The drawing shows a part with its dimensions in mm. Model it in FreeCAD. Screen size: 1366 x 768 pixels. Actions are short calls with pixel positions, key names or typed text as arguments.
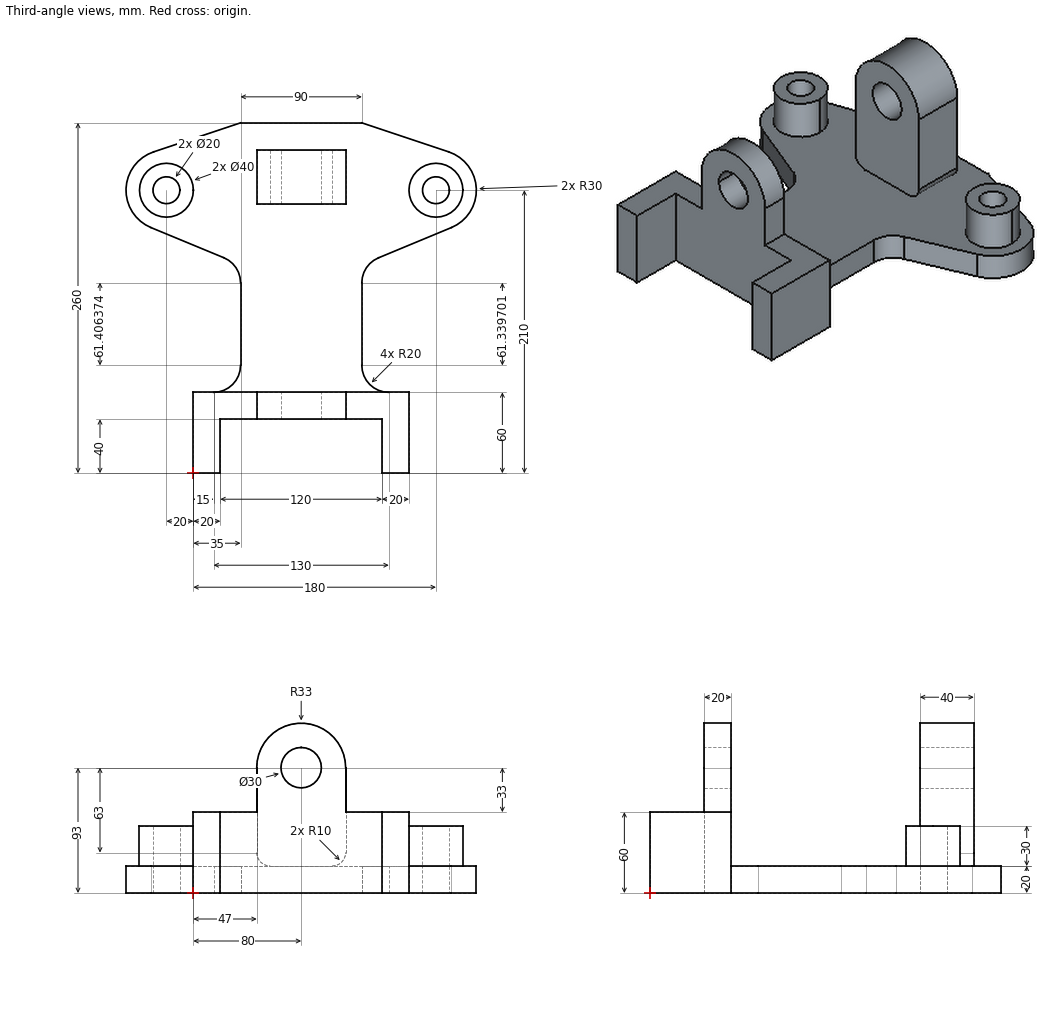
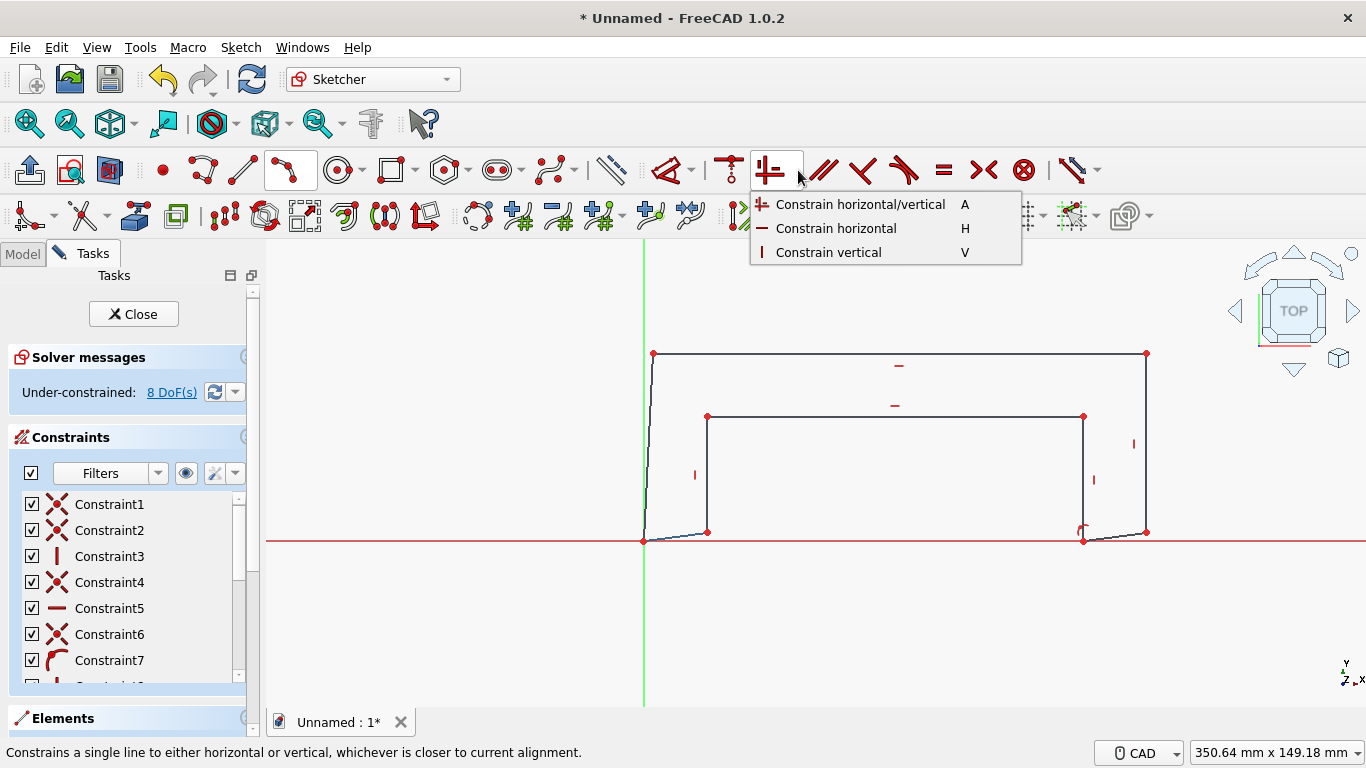
click(886, 228)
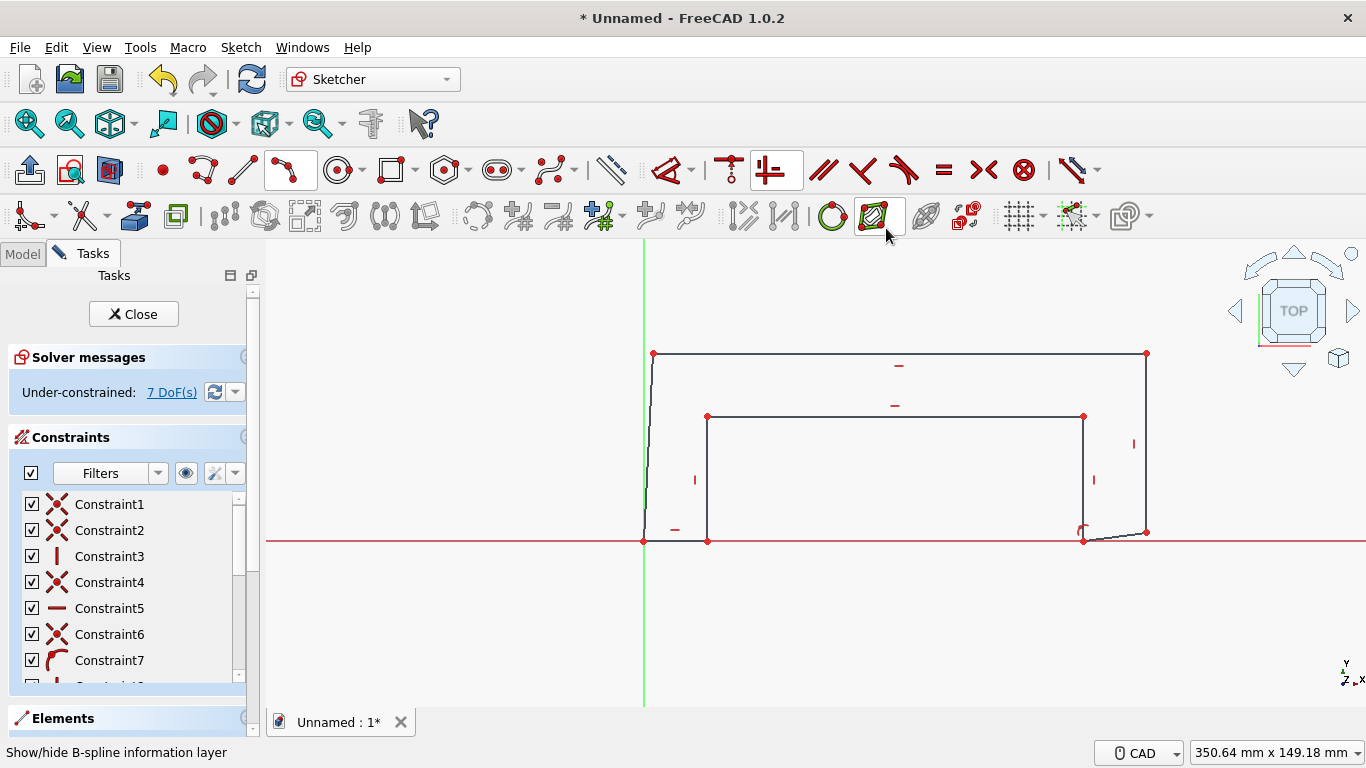
click(1102, 539)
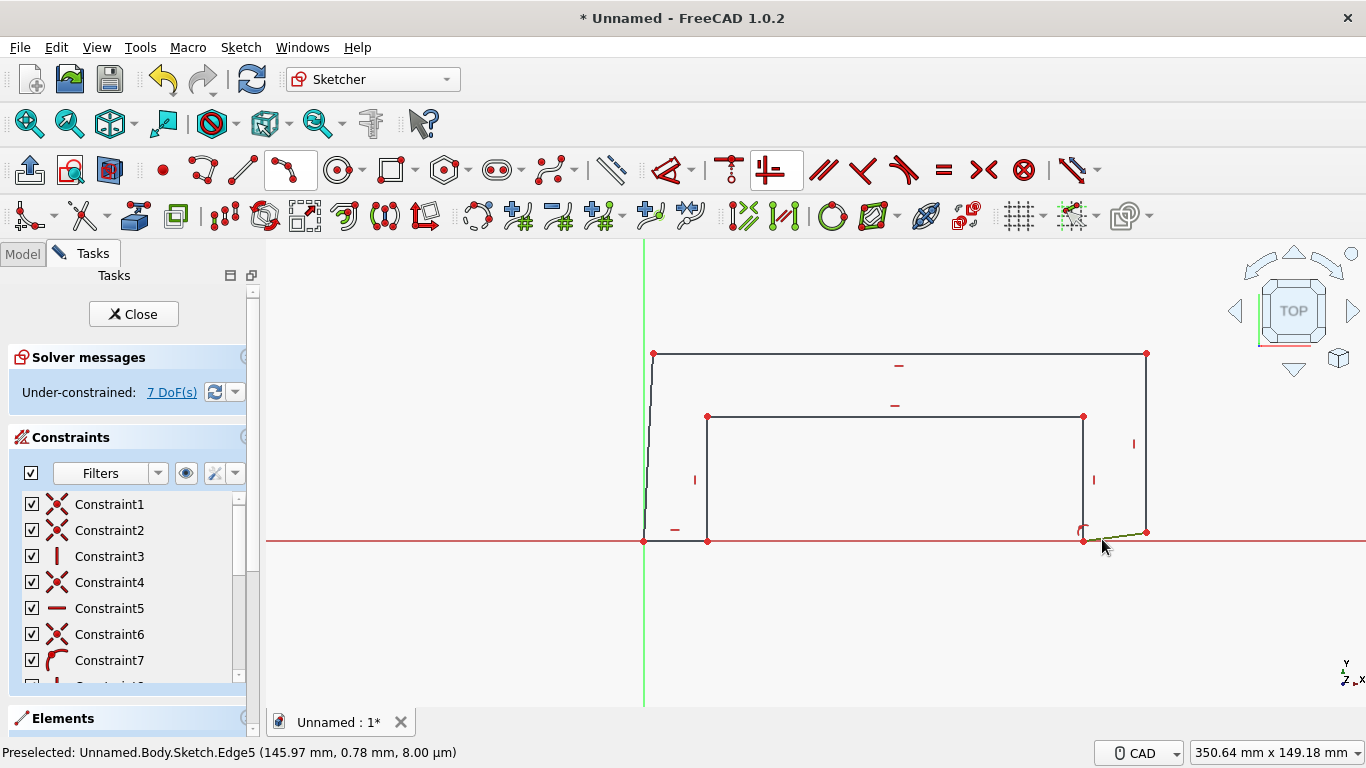
click(798, 170)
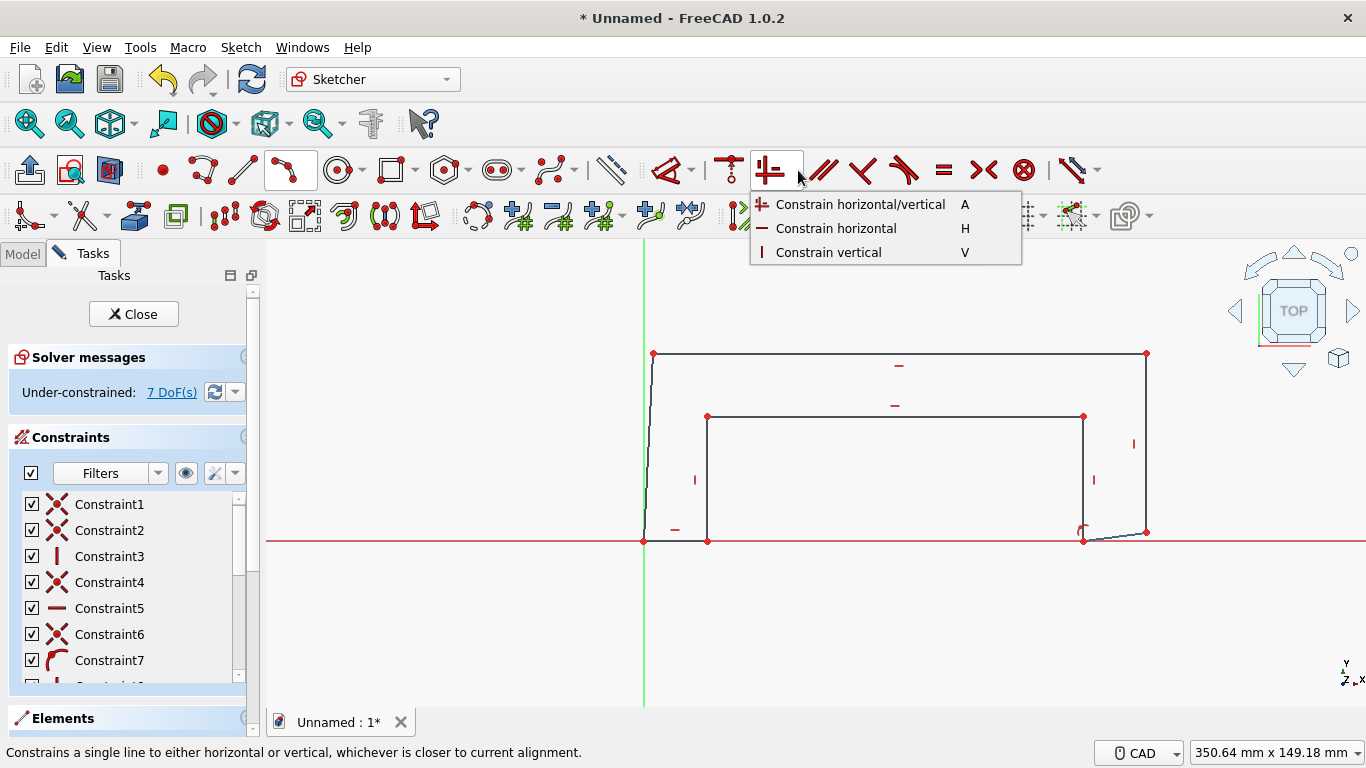
click(886, 228)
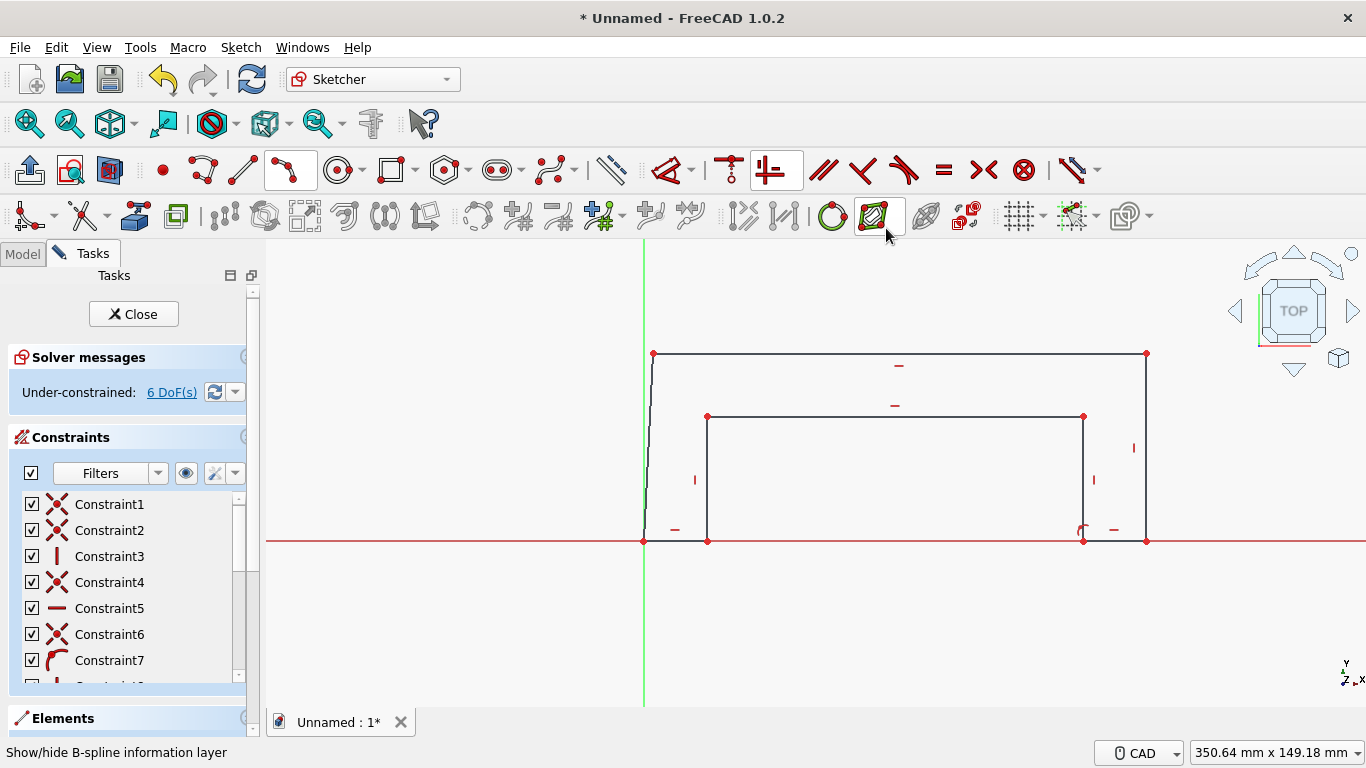
click(647, 485)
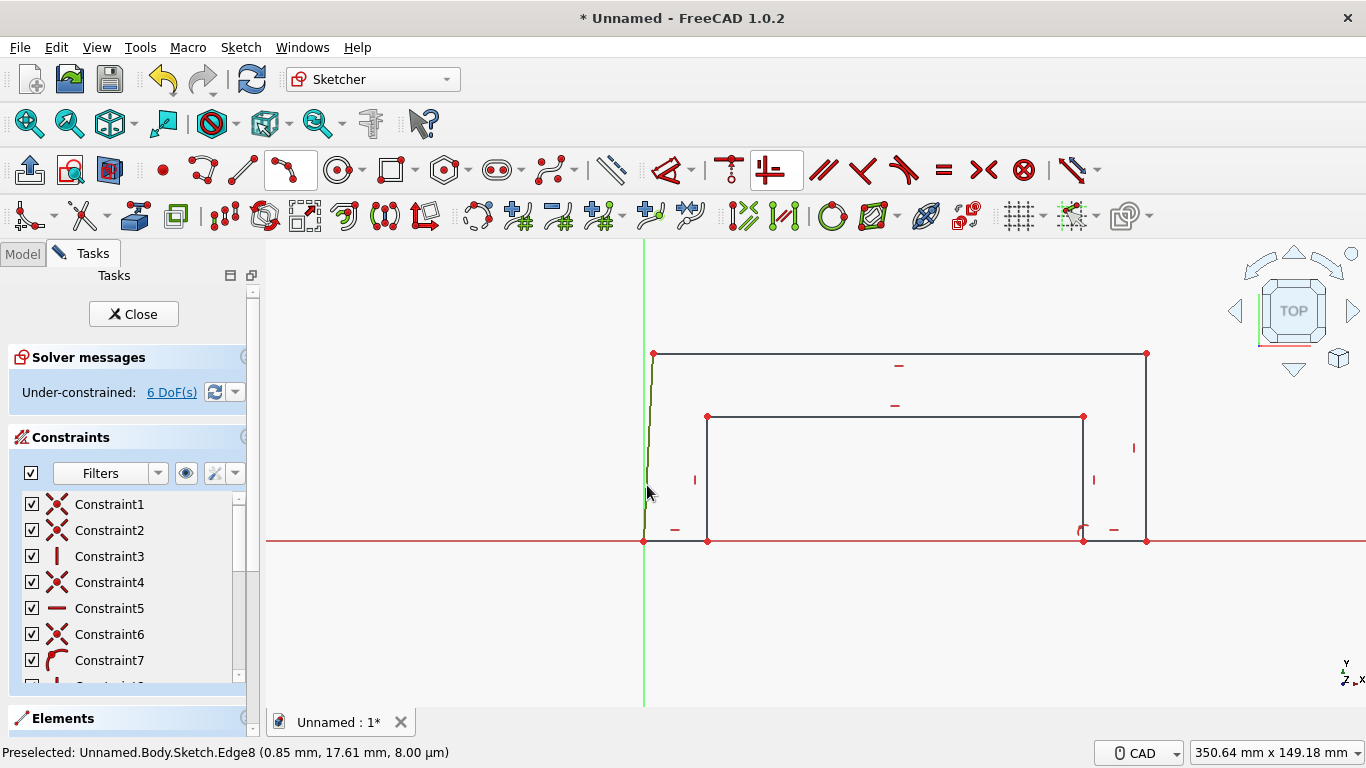
key(v)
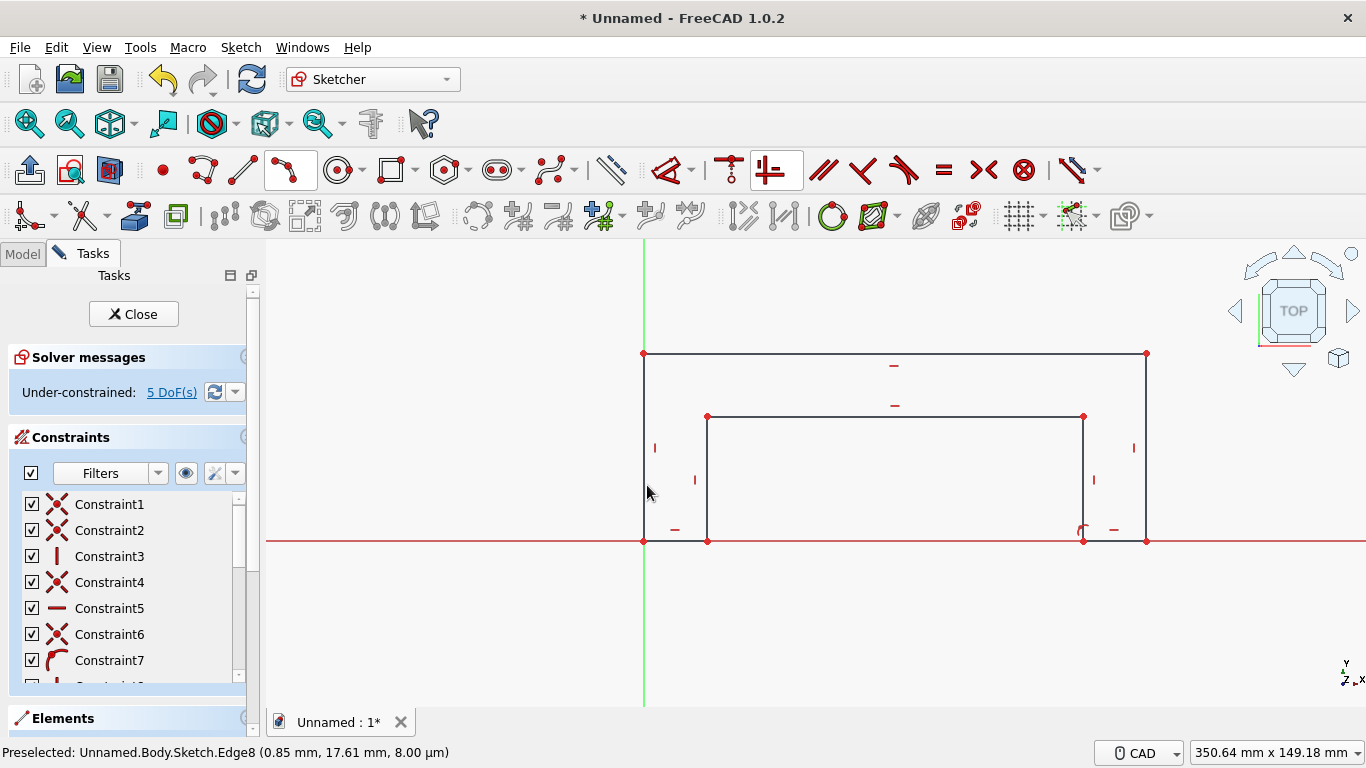
click(663, 541)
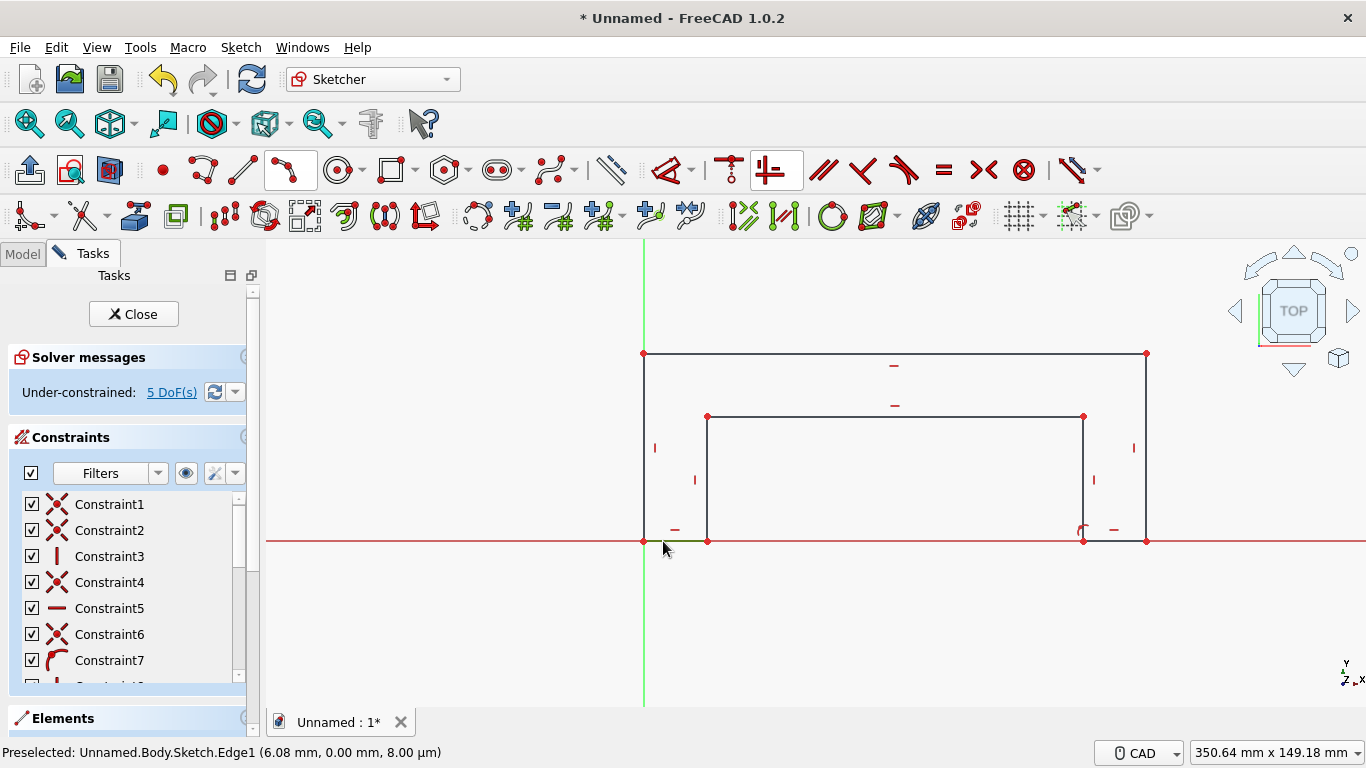
click(694, 170)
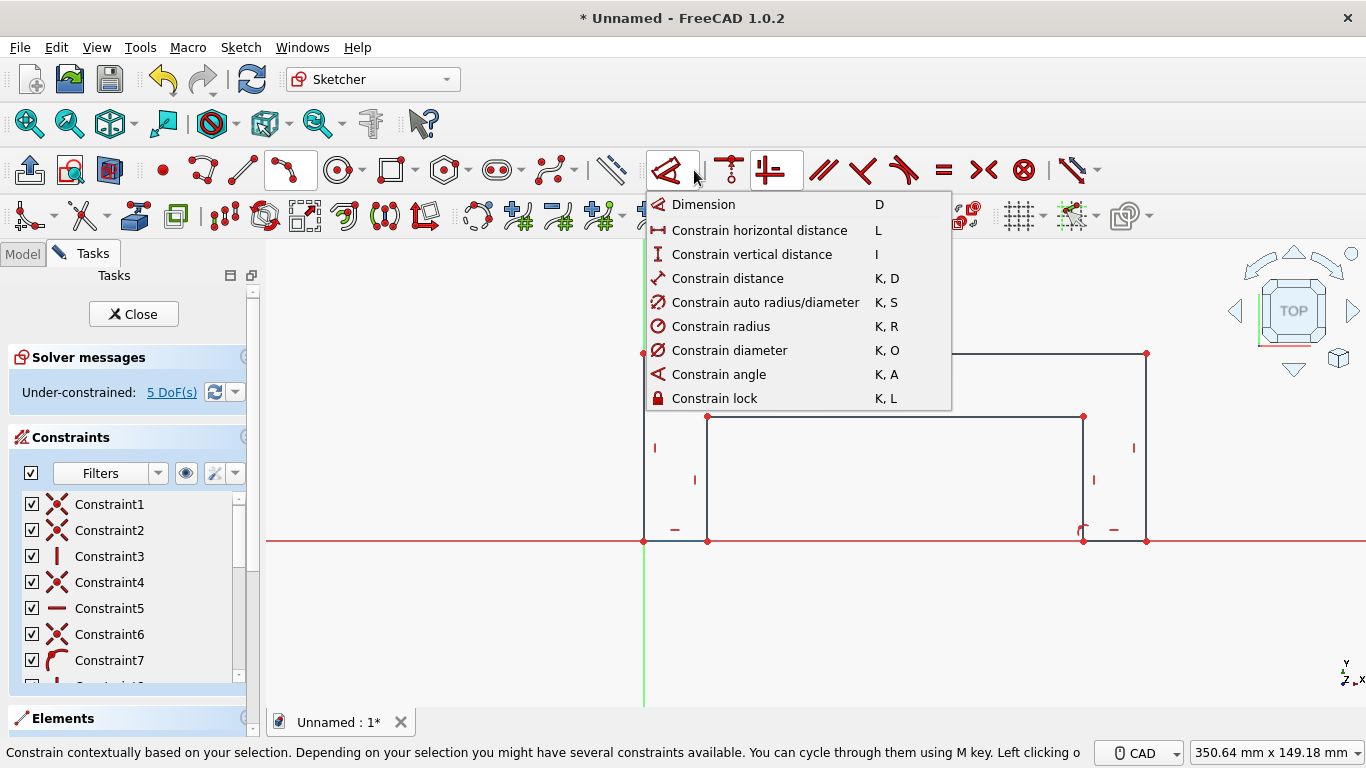
click(799, 230)